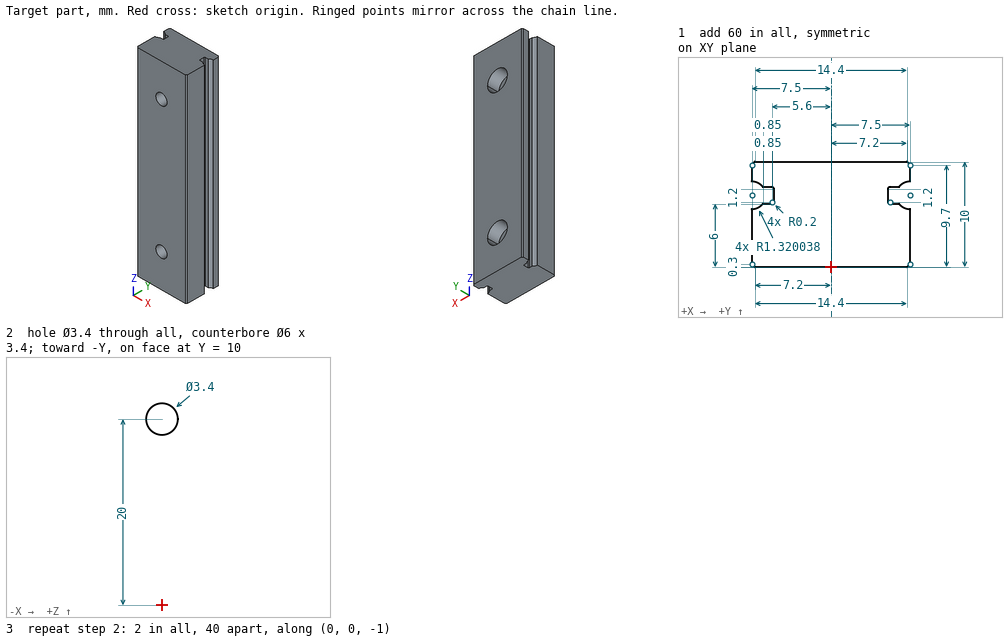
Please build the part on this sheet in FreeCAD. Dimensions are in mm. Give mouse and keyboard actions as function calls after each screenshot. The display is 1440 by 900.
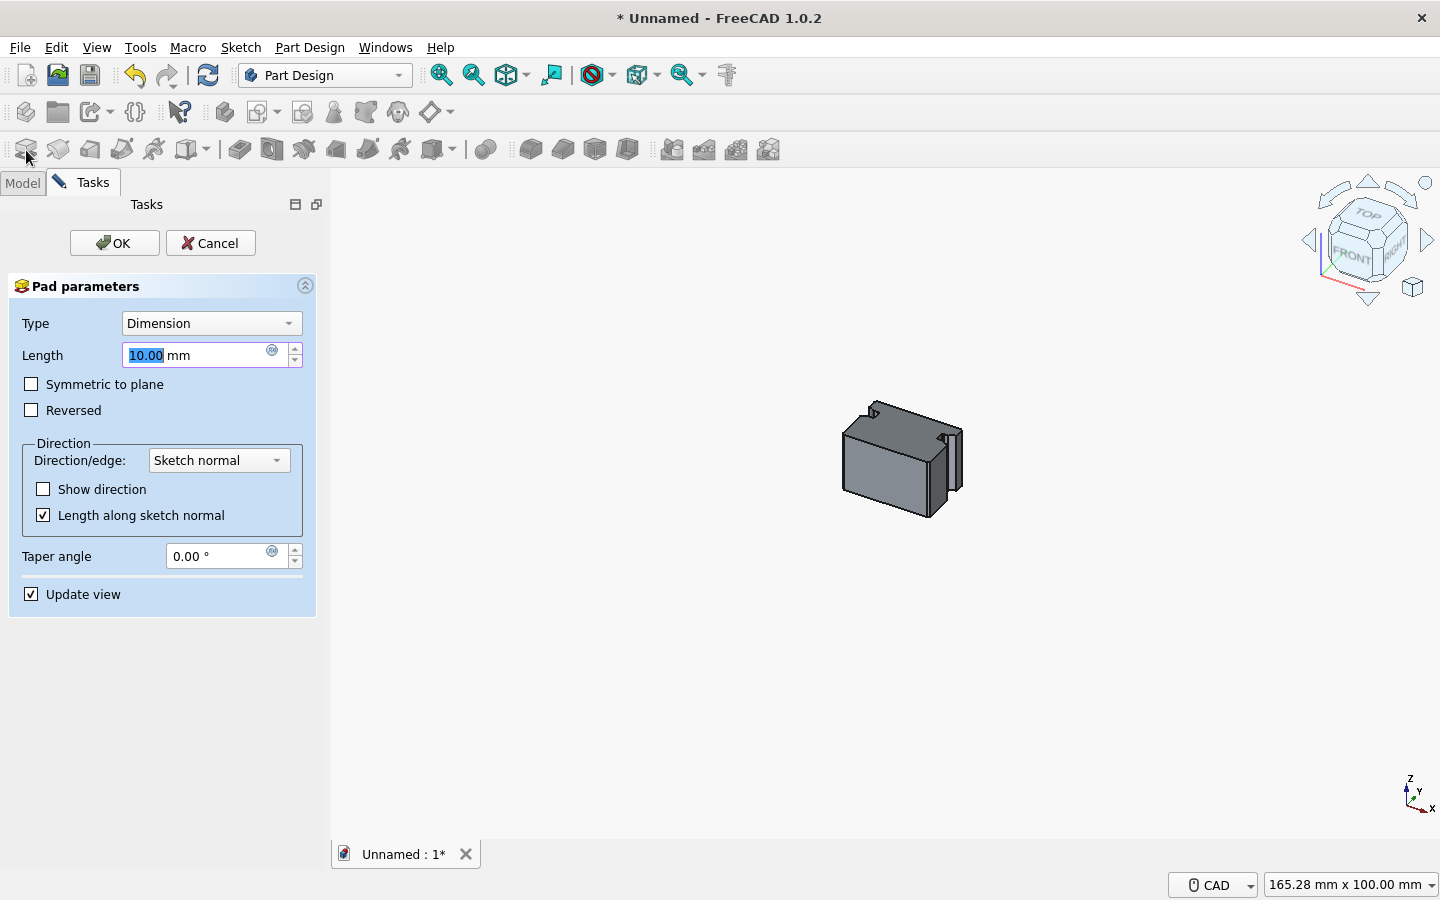
text(60)
key(Tab)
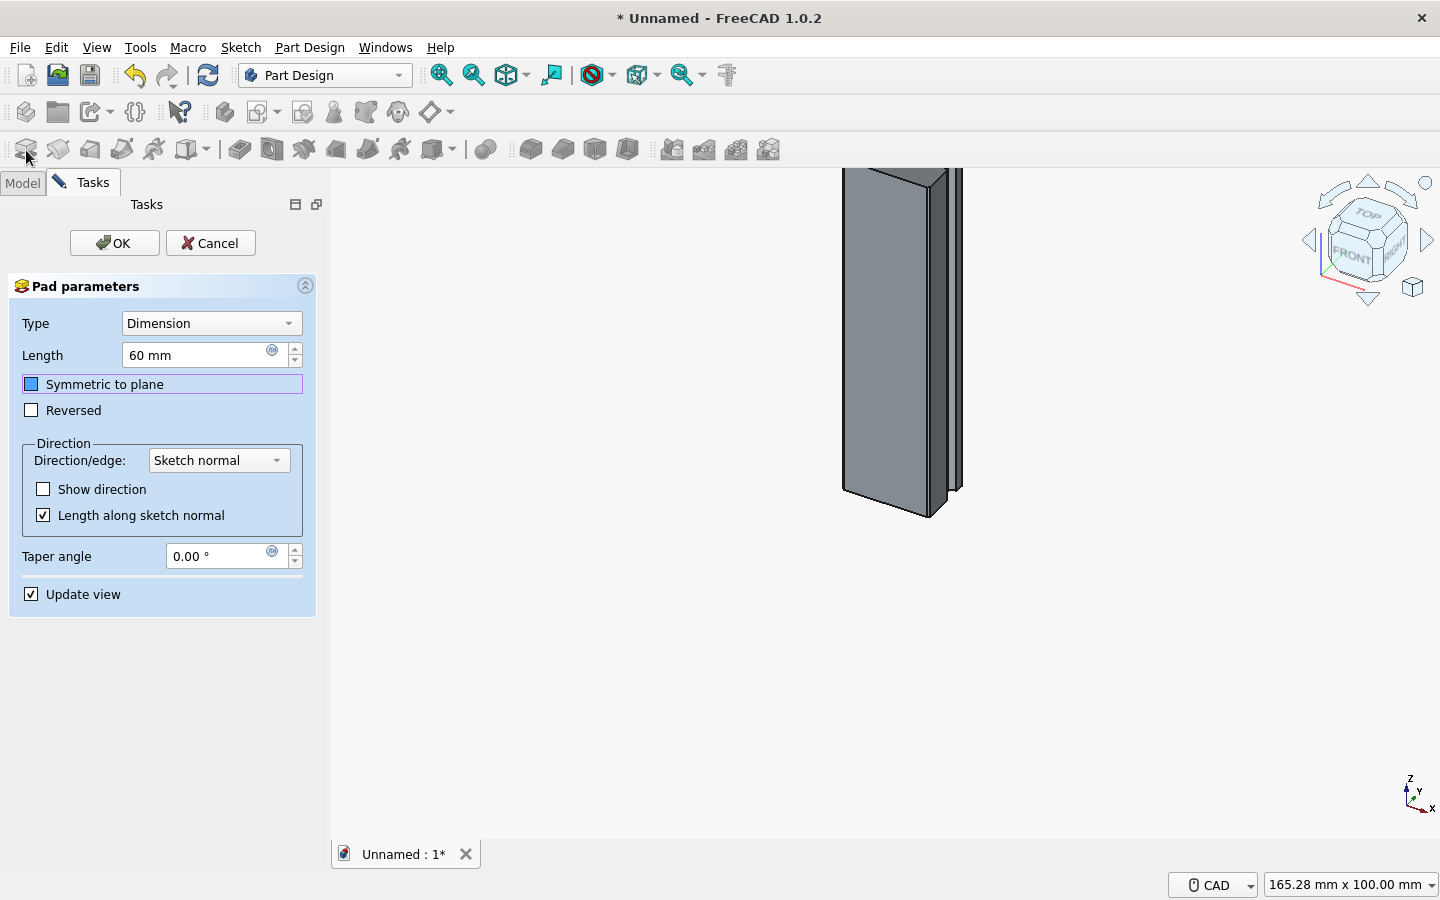
click(30, 384)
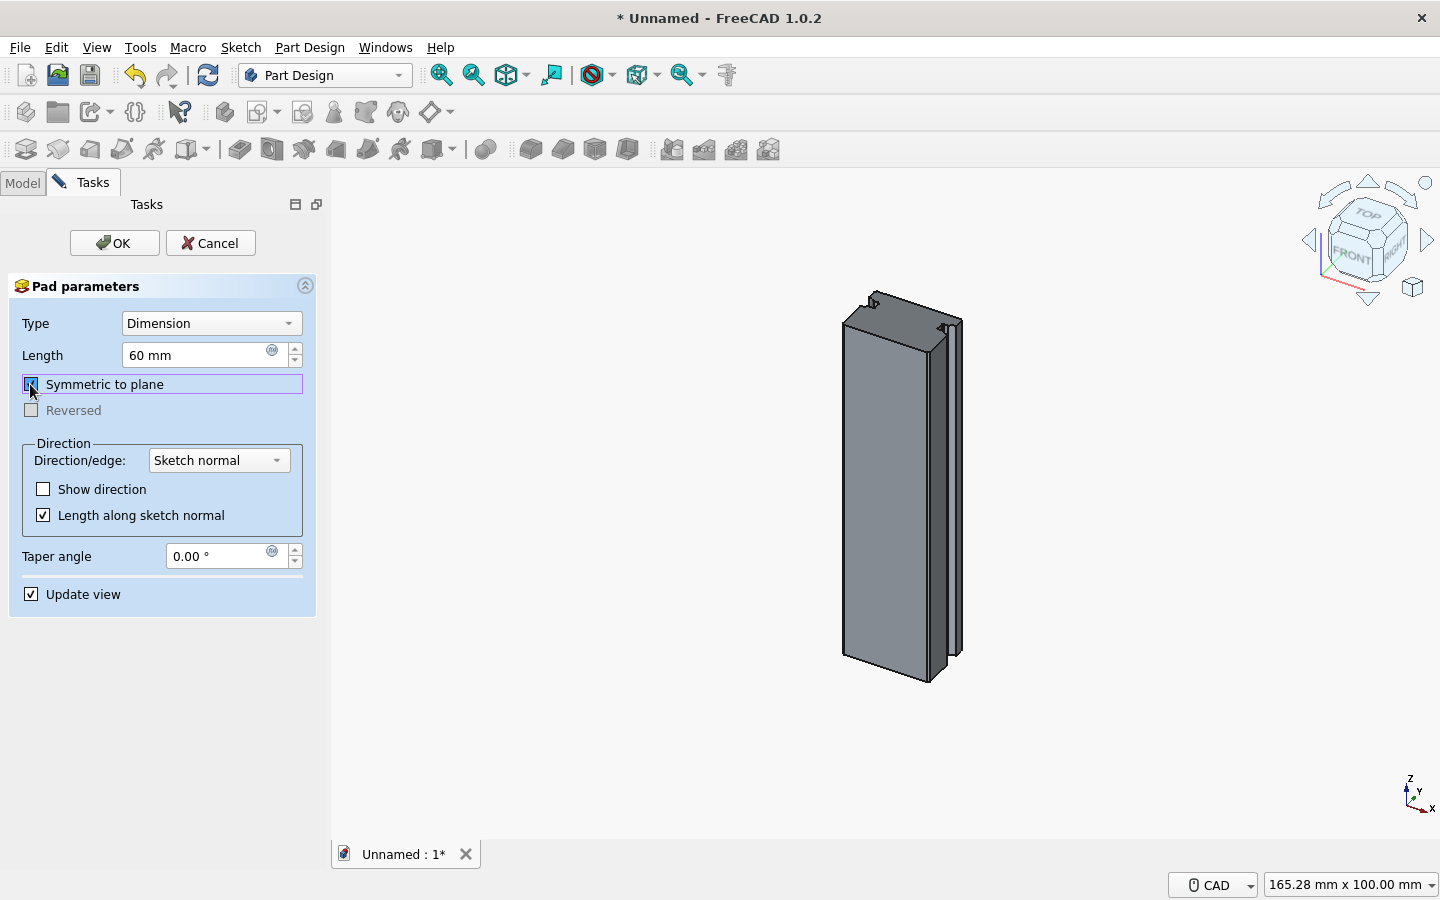
click(115, 243)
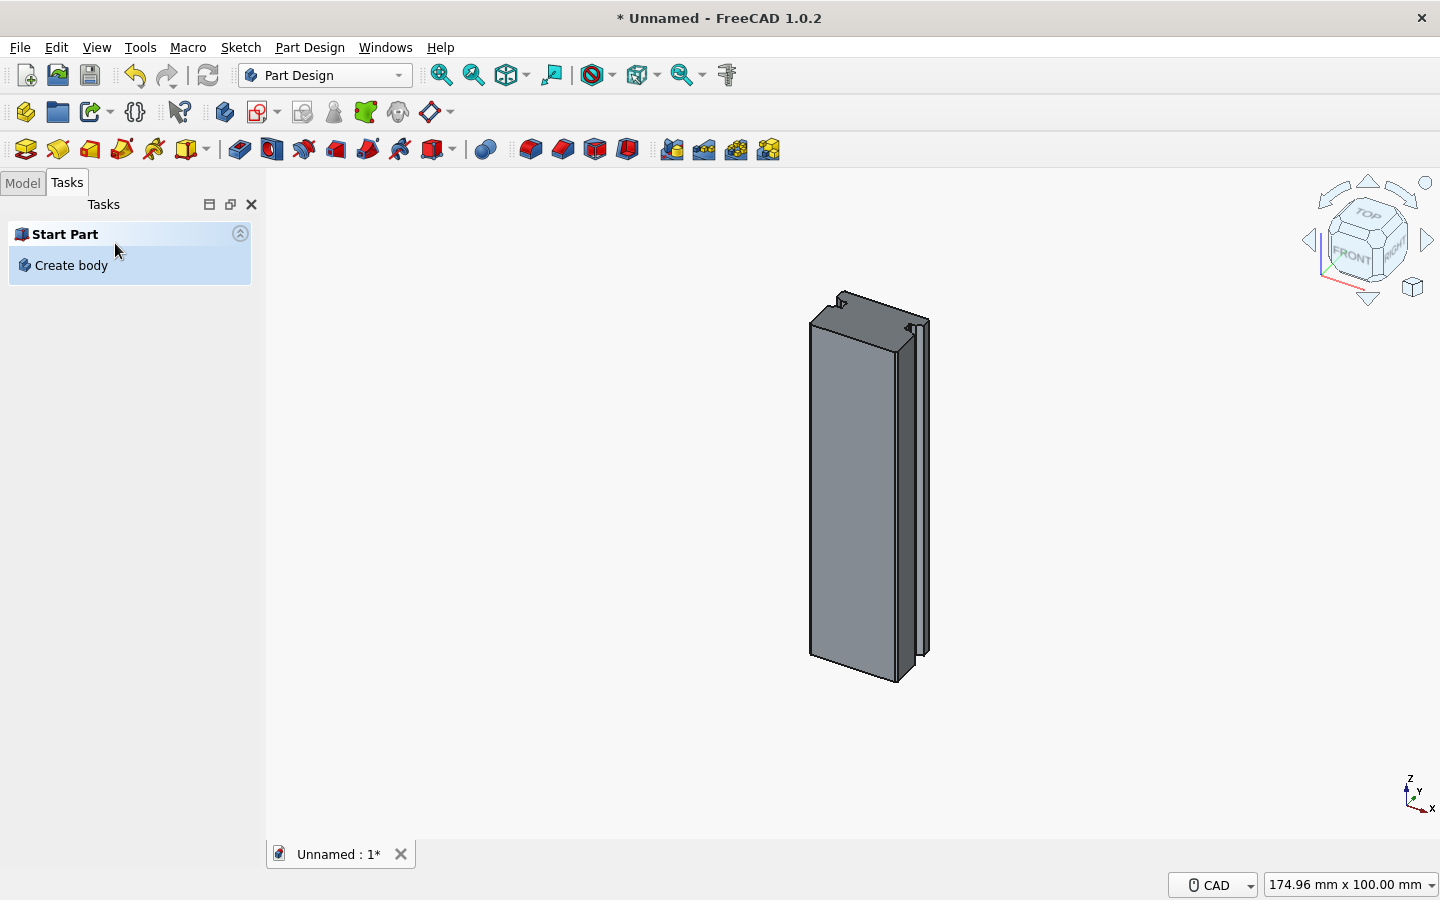
key(4)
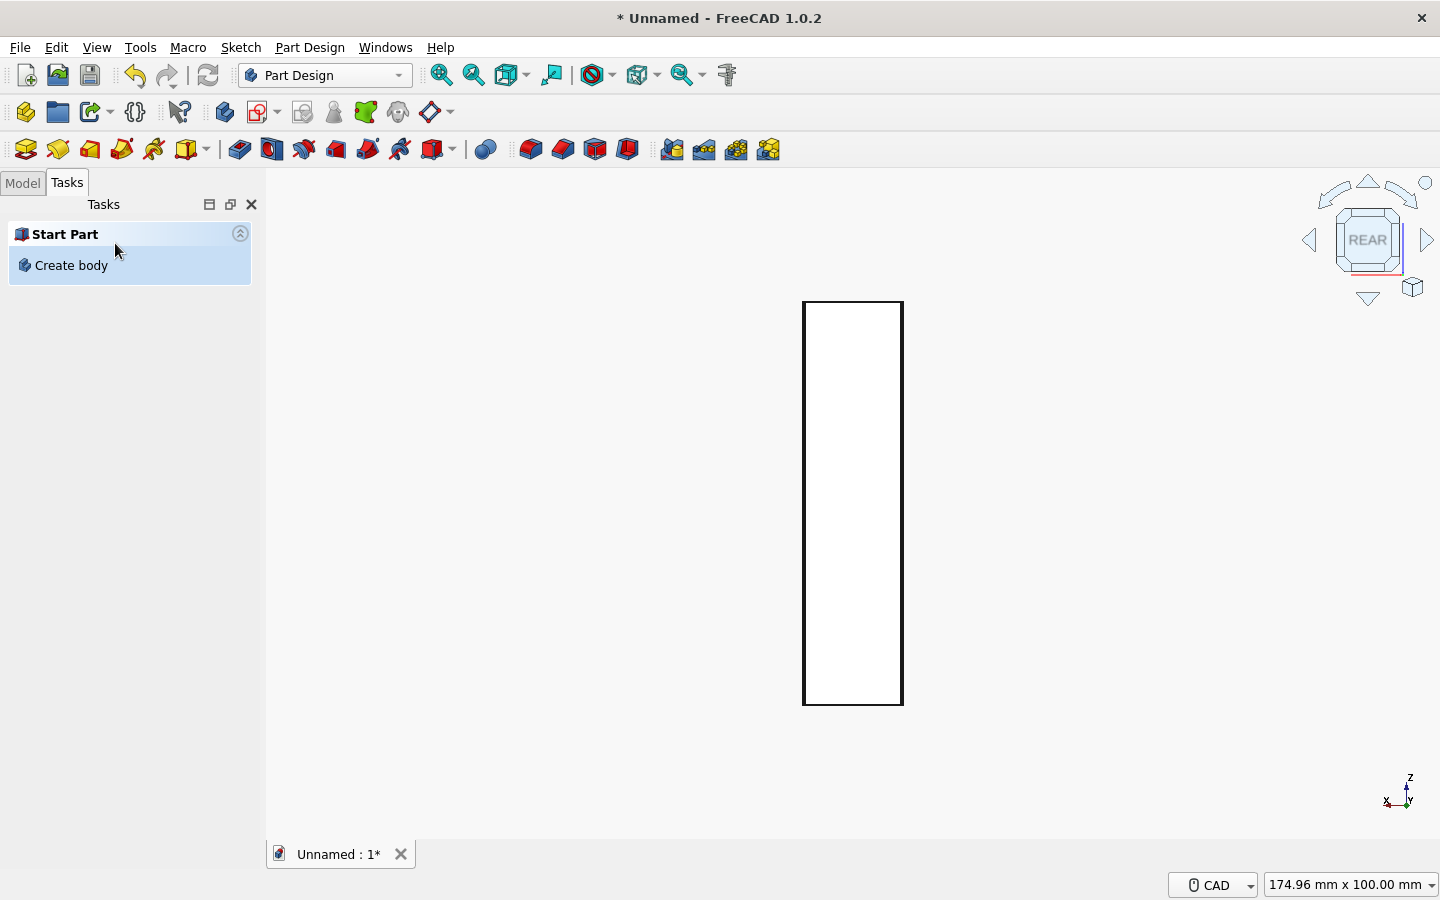
click(853, 387)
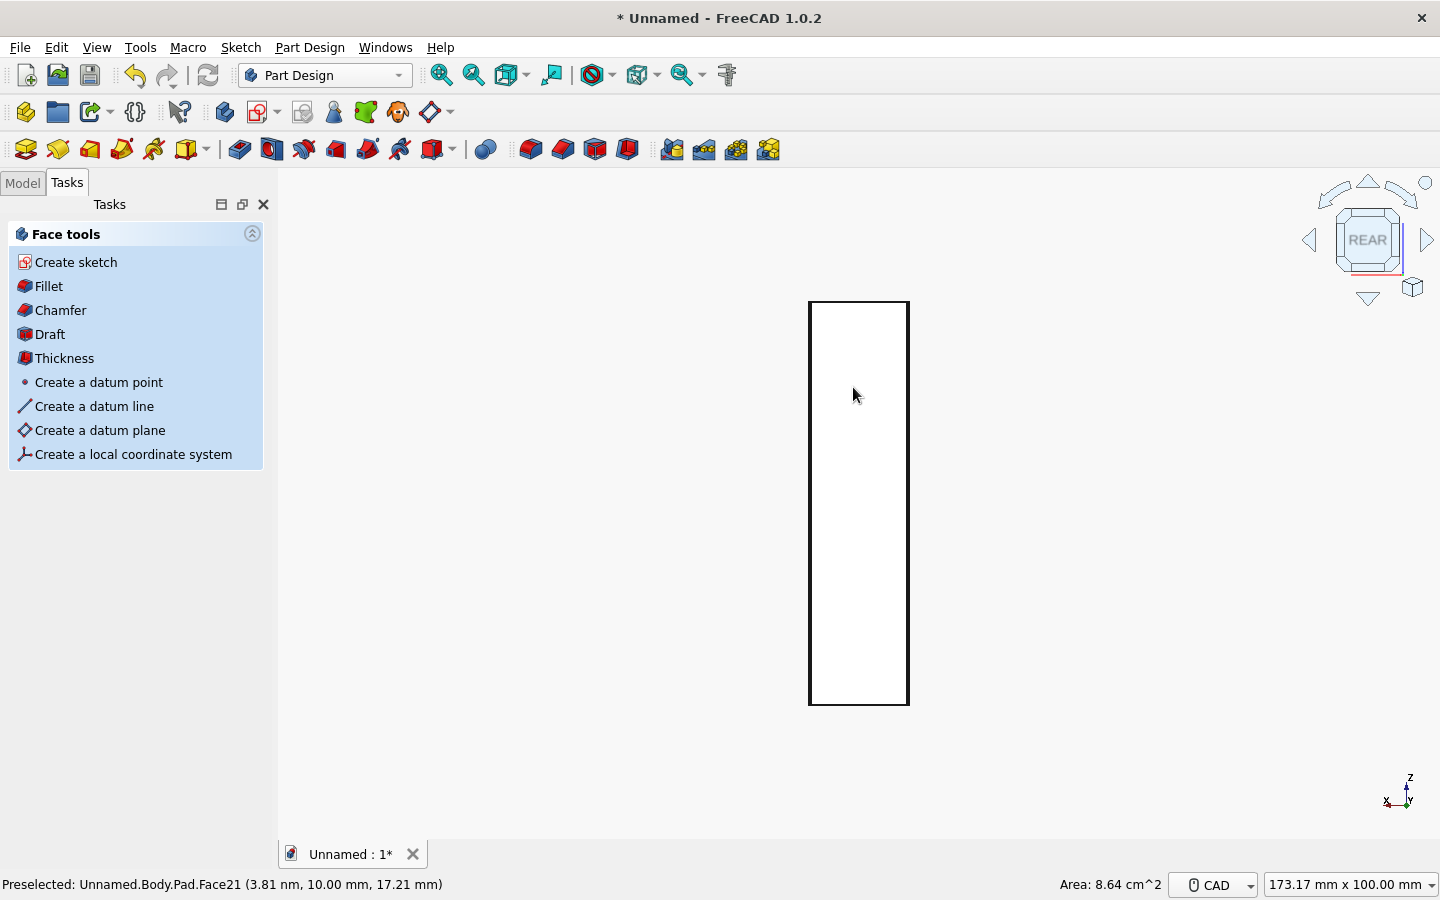
click(258, 112)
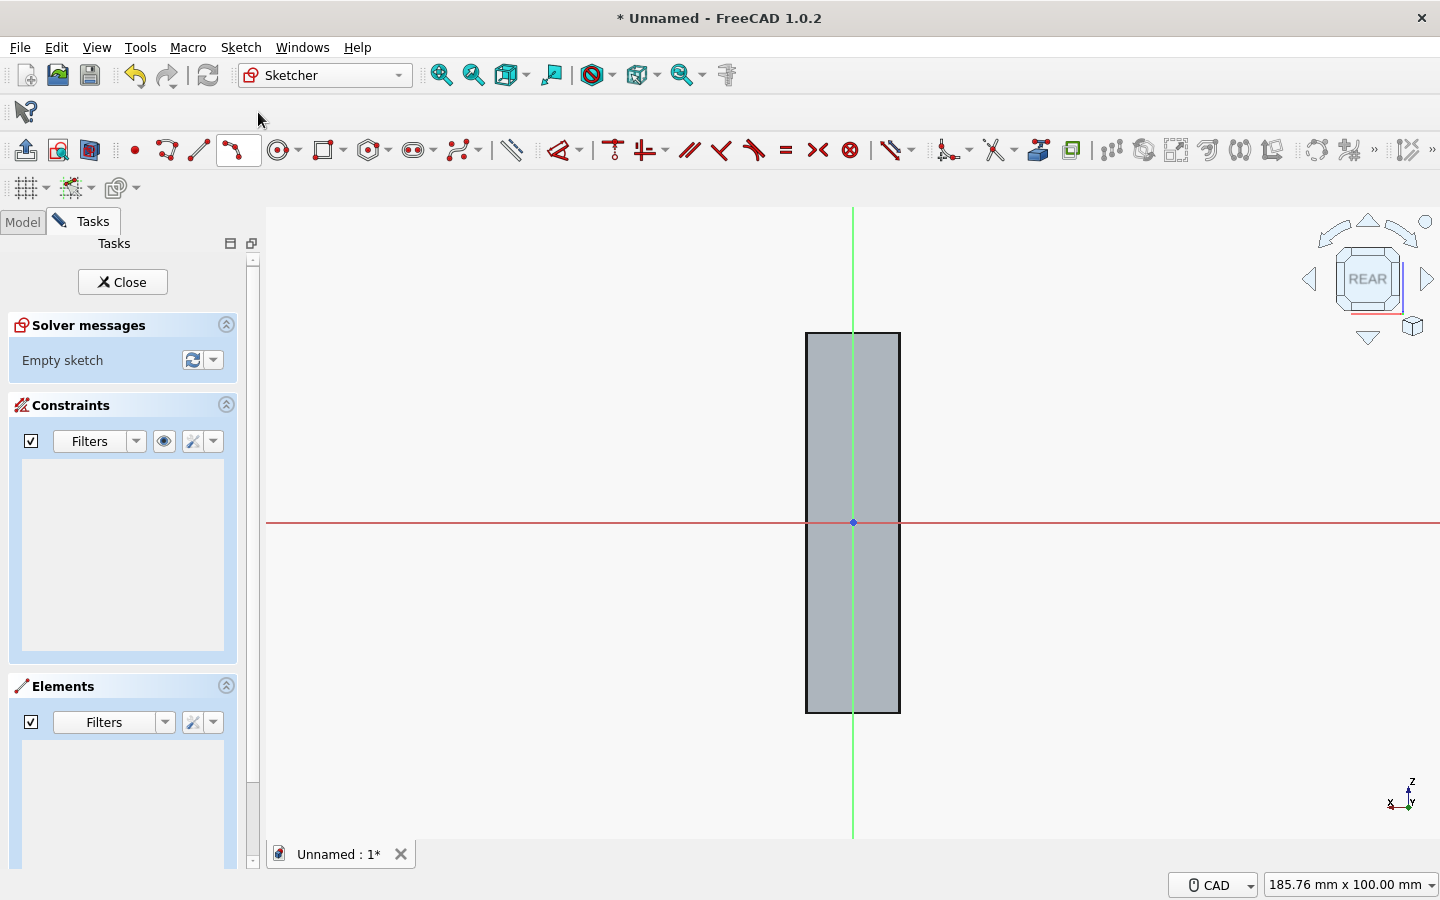
scroll(857, 390, up, 15)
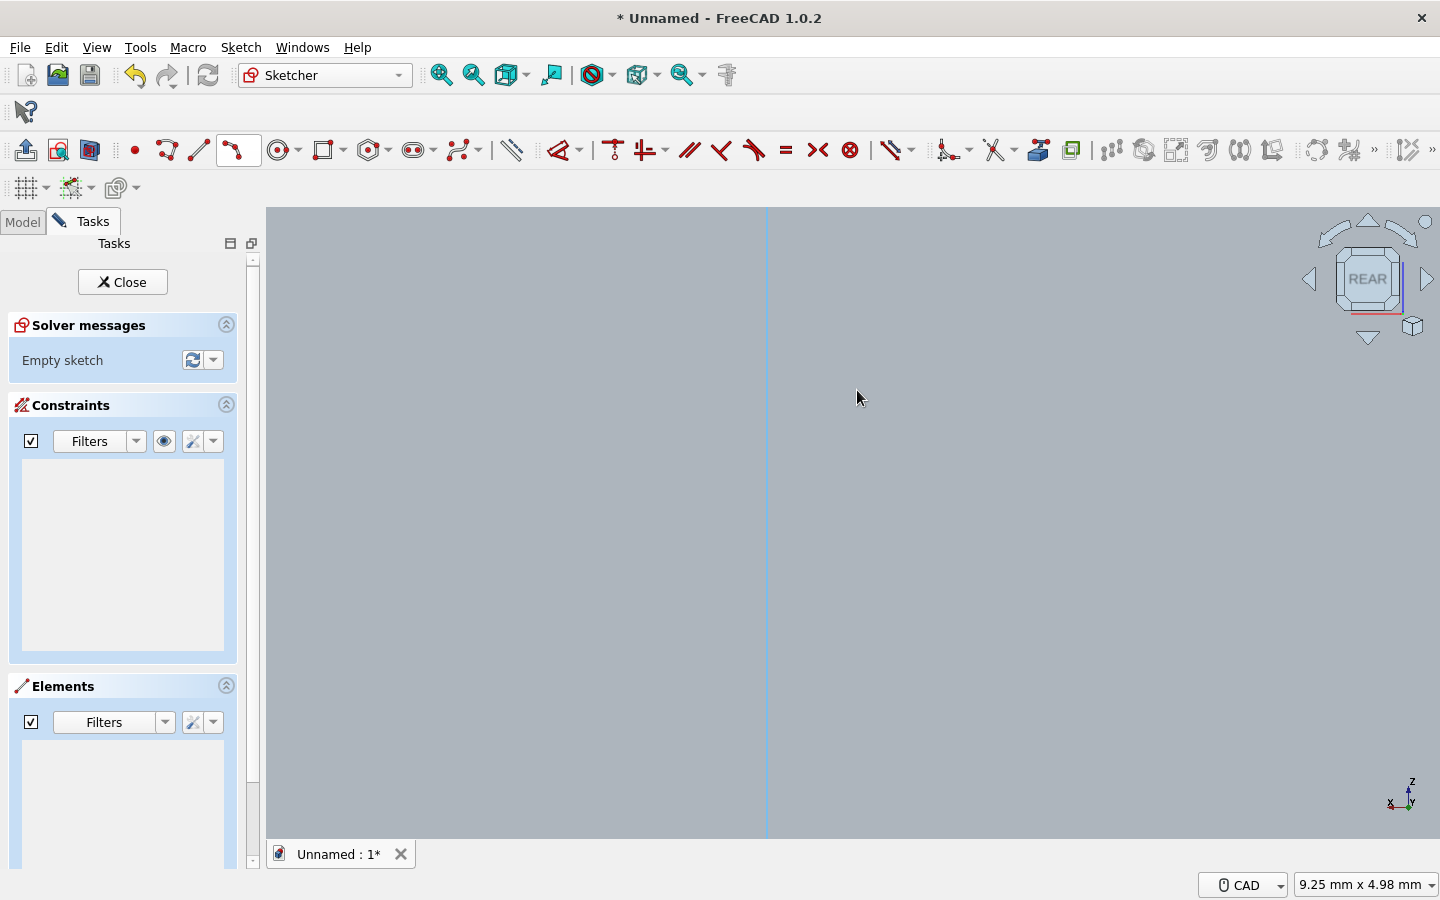
key(g)
key(c)